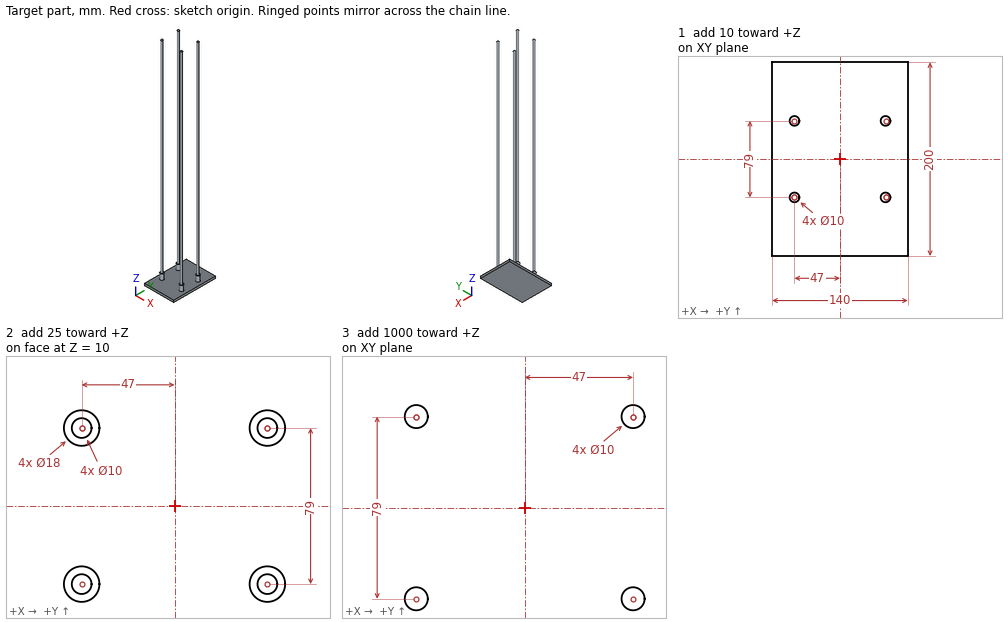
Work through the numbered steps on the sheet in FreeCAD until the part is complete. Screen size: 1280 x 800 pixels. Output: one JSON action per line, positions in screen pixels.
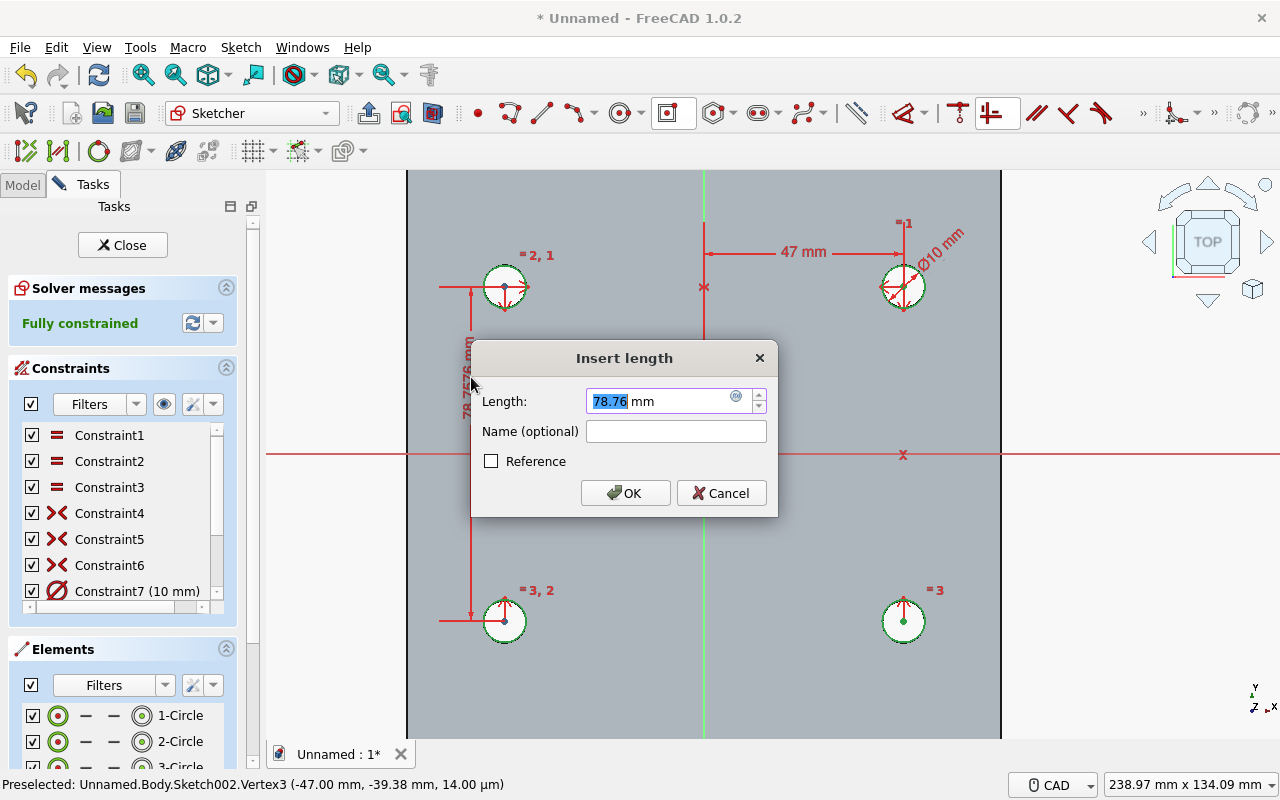
{"action": "type", "text": "79"}
{"action": "key", "text": "Return"}
{"action": "key", "text": "Escape"}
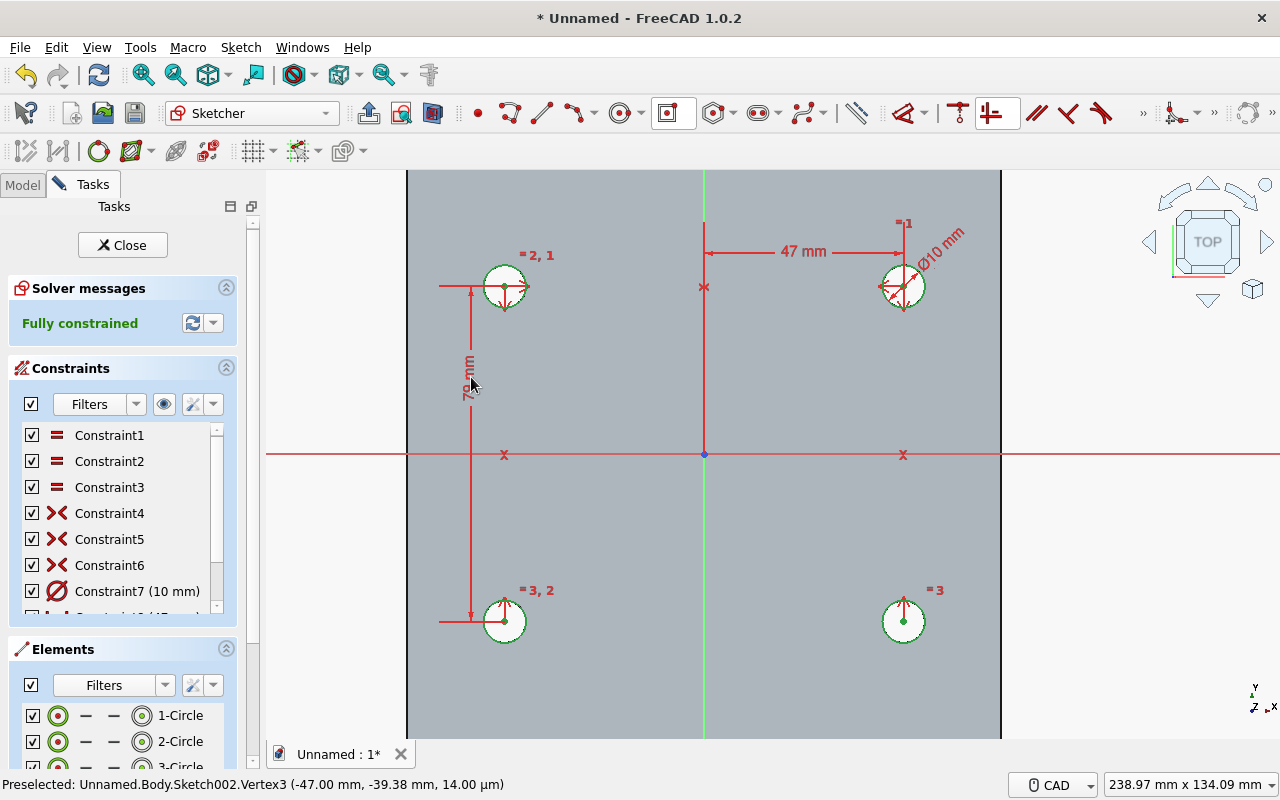
{"action": "left_click", "coordinate": [123, 245]}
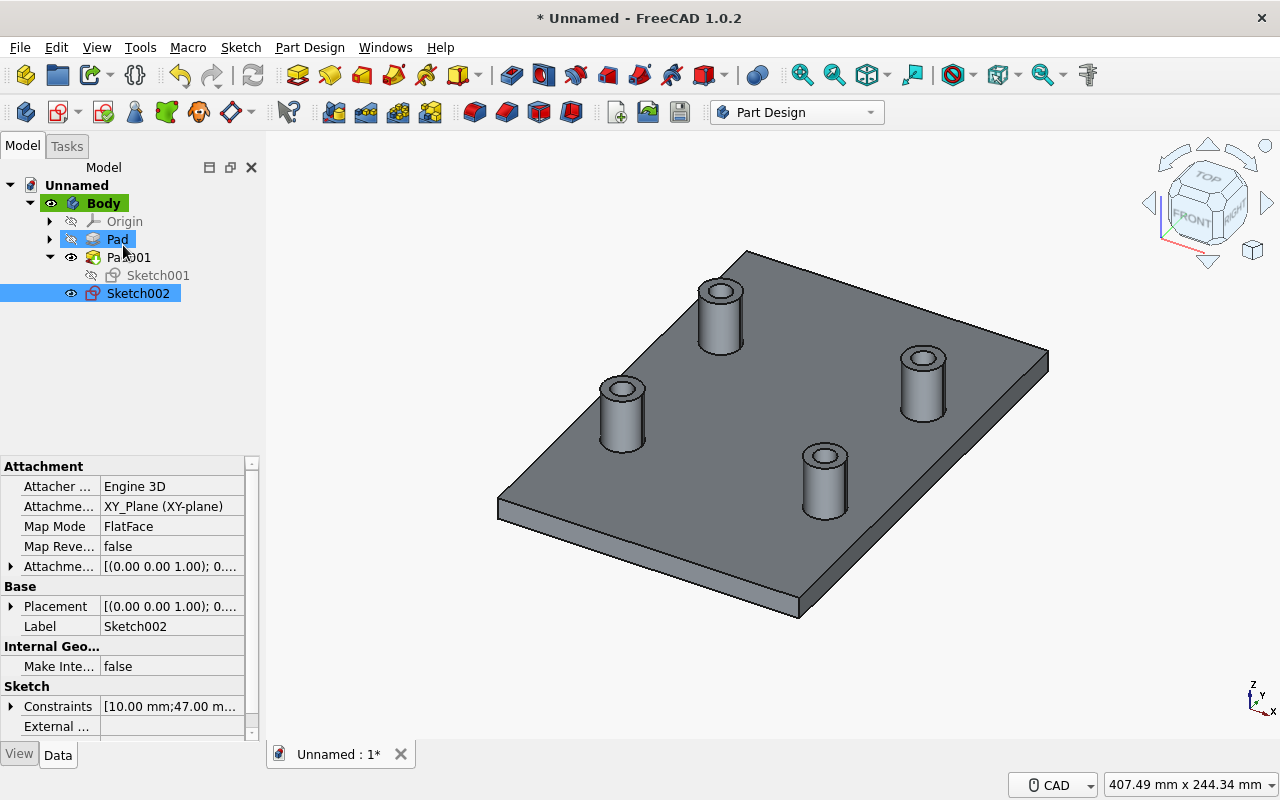
{"action": "left_click", "coordinate": [298, 76]}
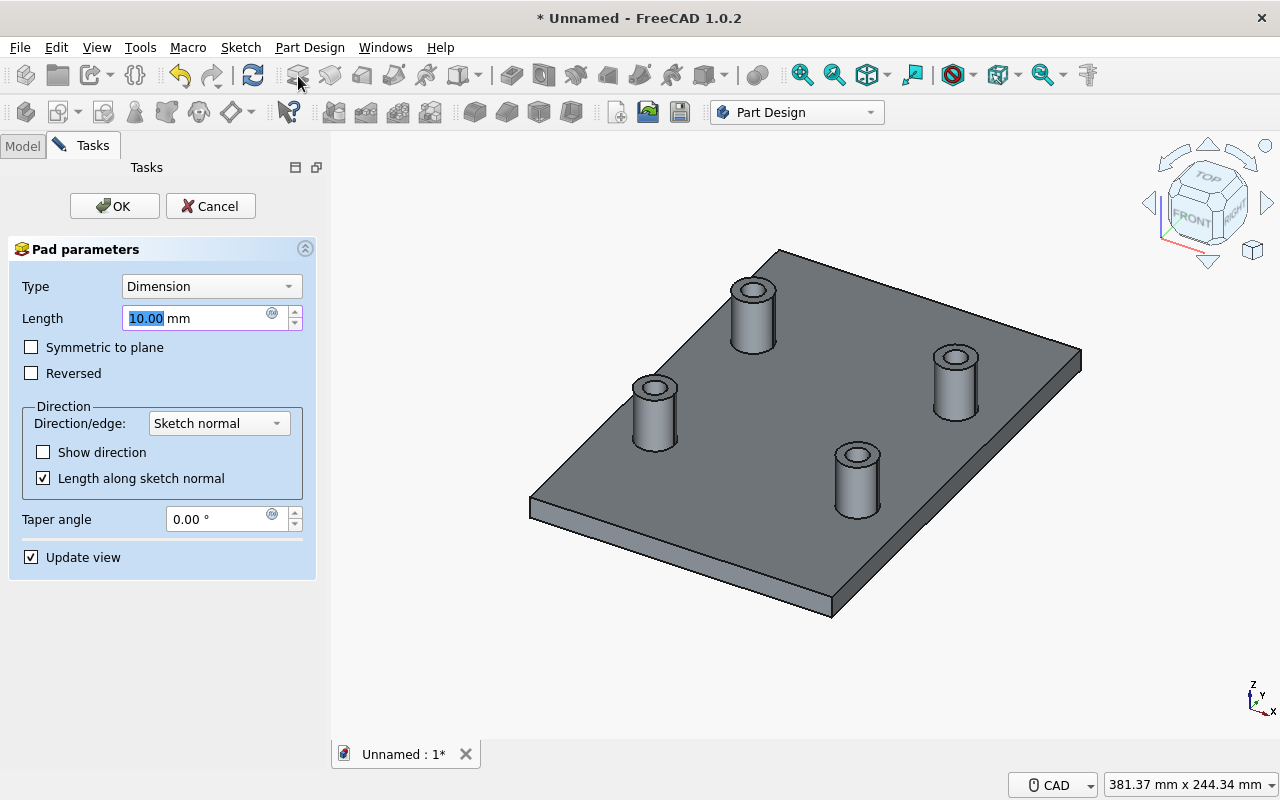
{"action": "type", "text": "1000"}
{"action": "key", "text": "Tab"}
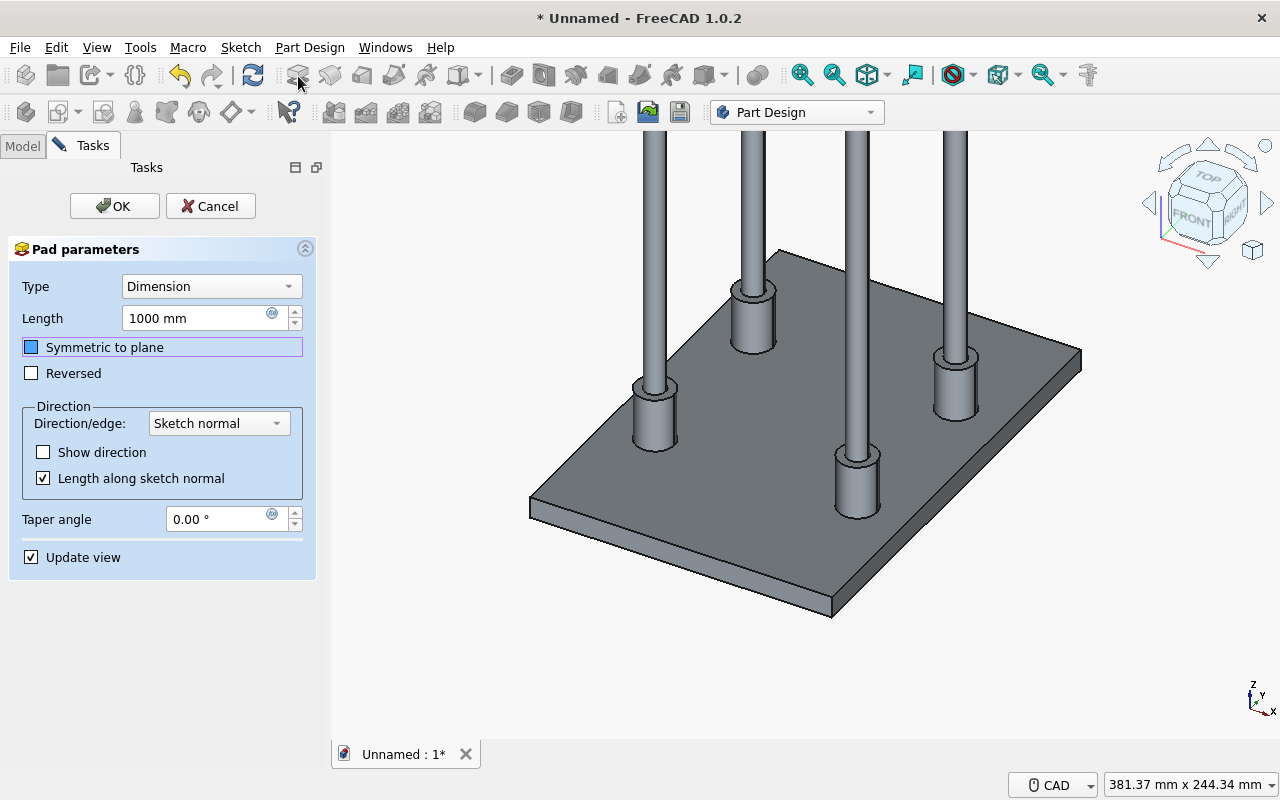
{"action": "left_click", "coordinate": [115, 206]}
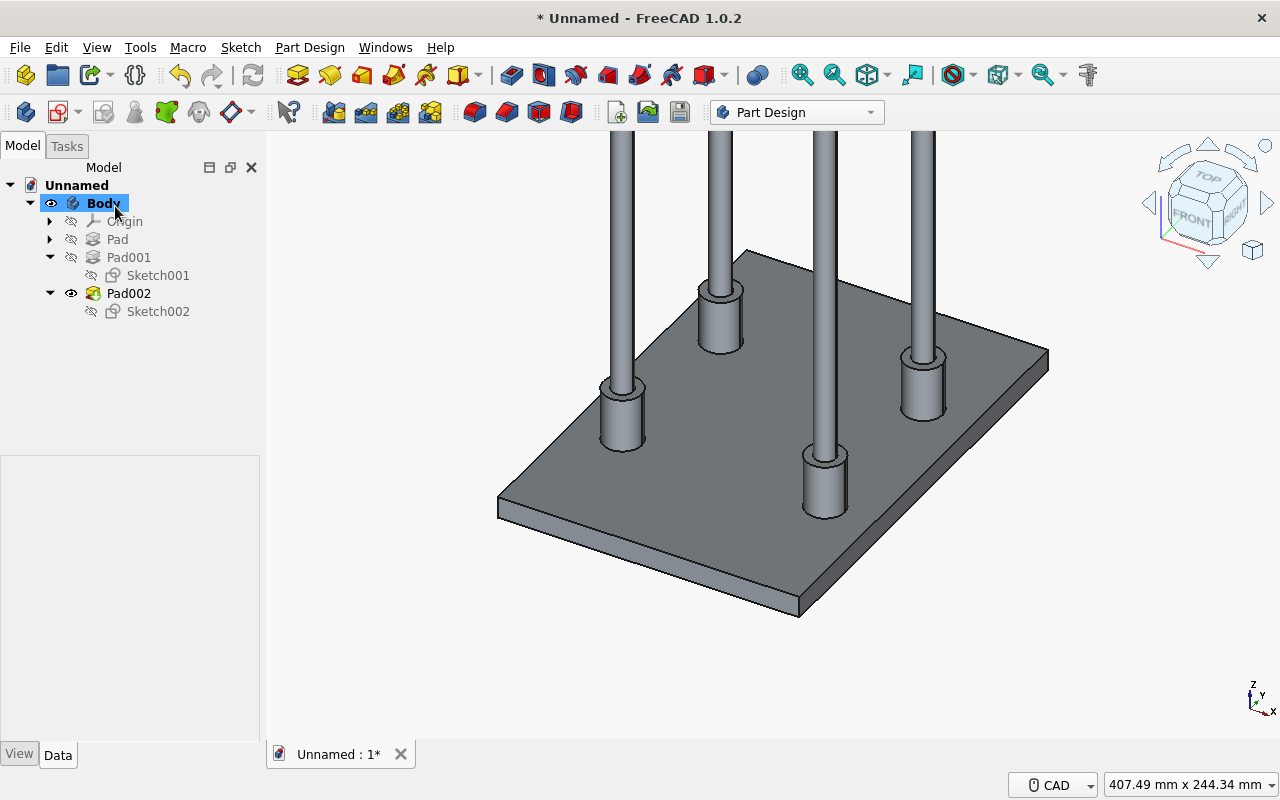
{"action": "key", "text": "0"}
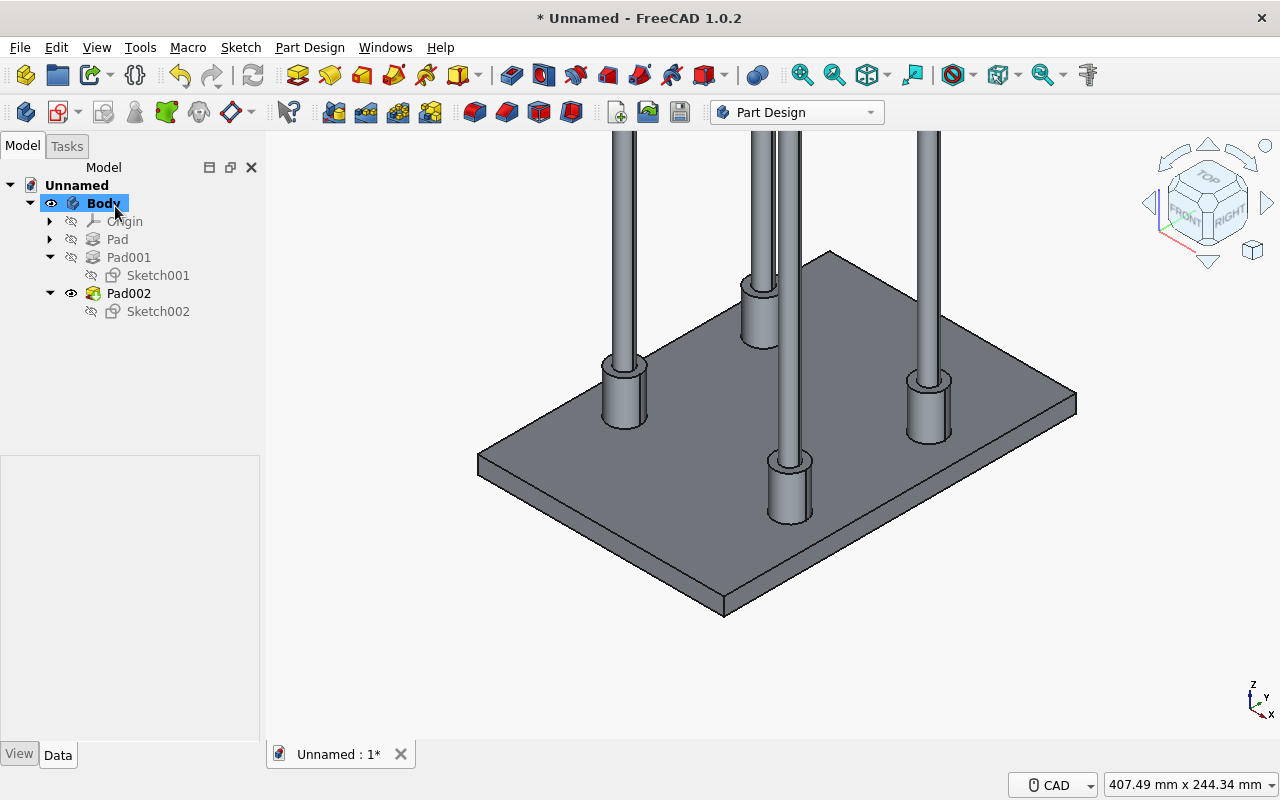
{"action": "left_click", "coordinate": [804, 76]}